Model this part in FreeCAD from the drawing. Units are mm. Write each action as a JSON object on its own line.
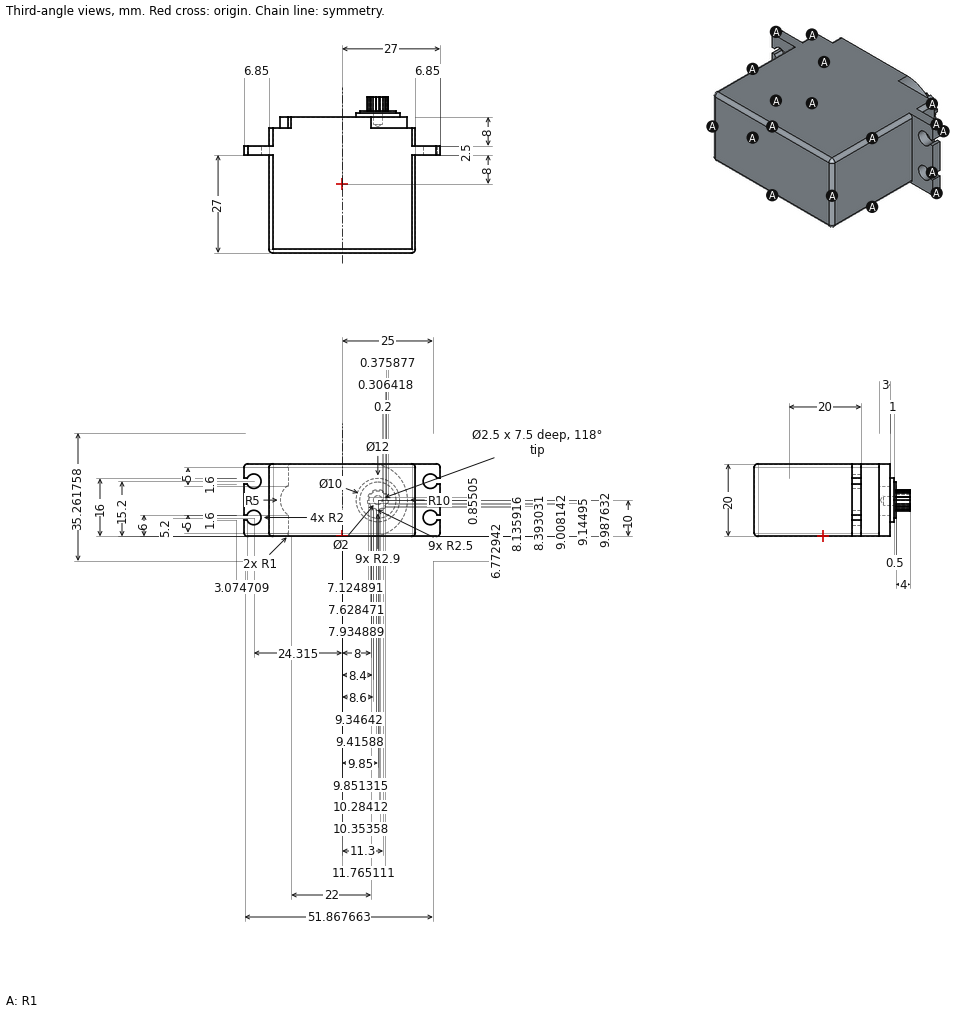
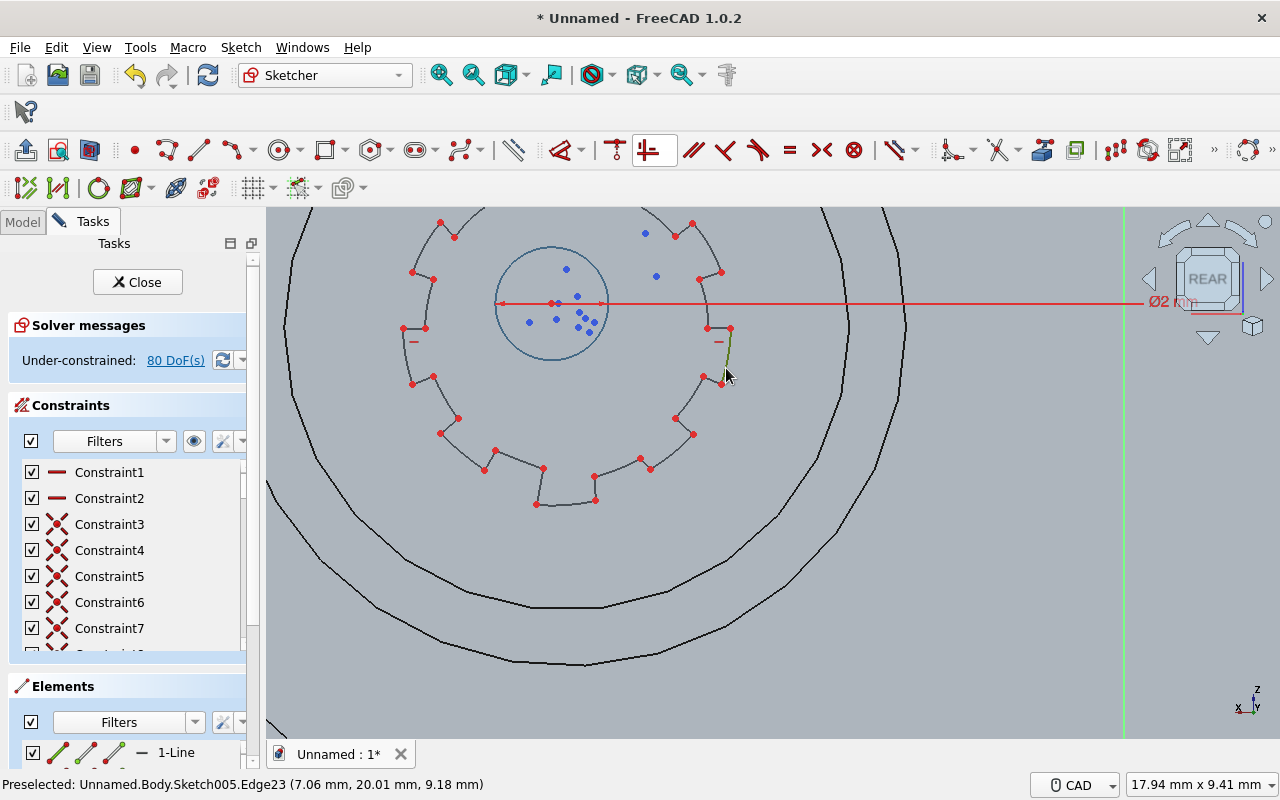
{"action": "left_click", "coordinate": [616, 150]}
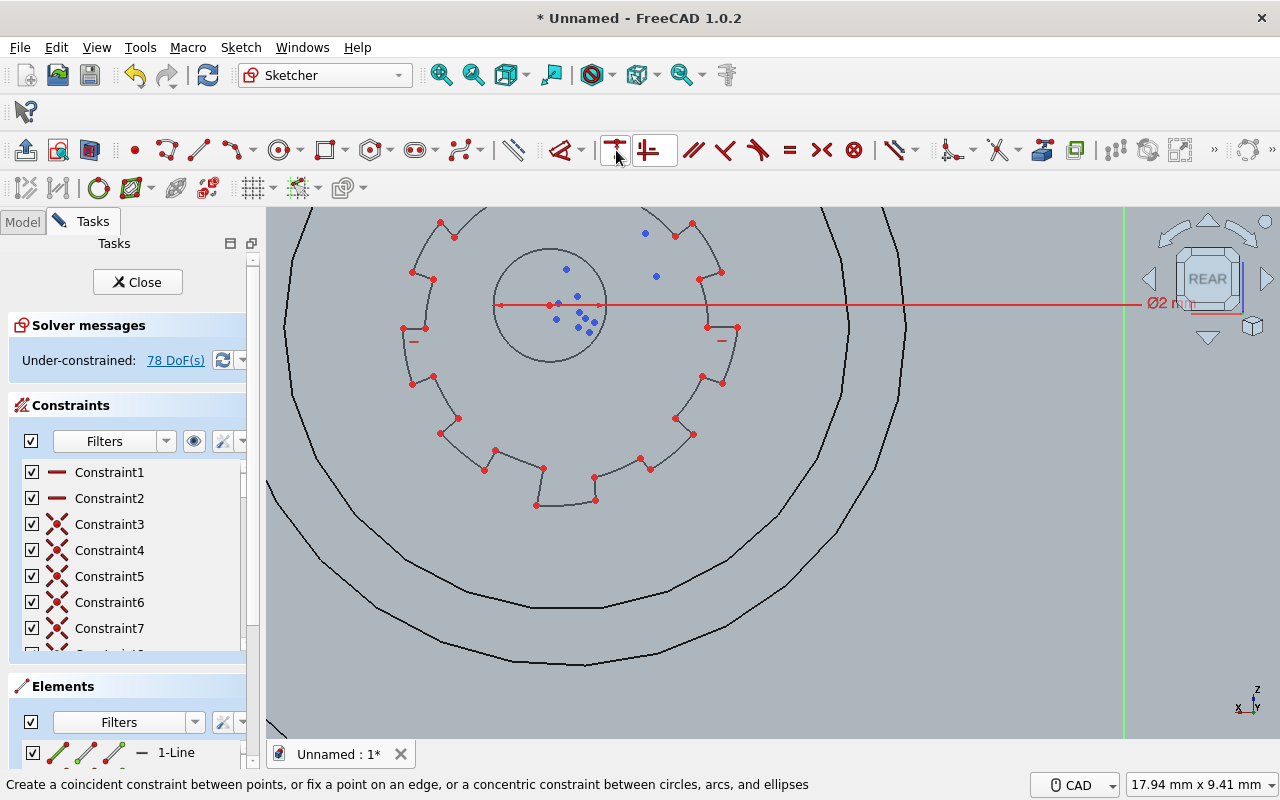
{"action": "left_click", "coordinate": [590, 265]}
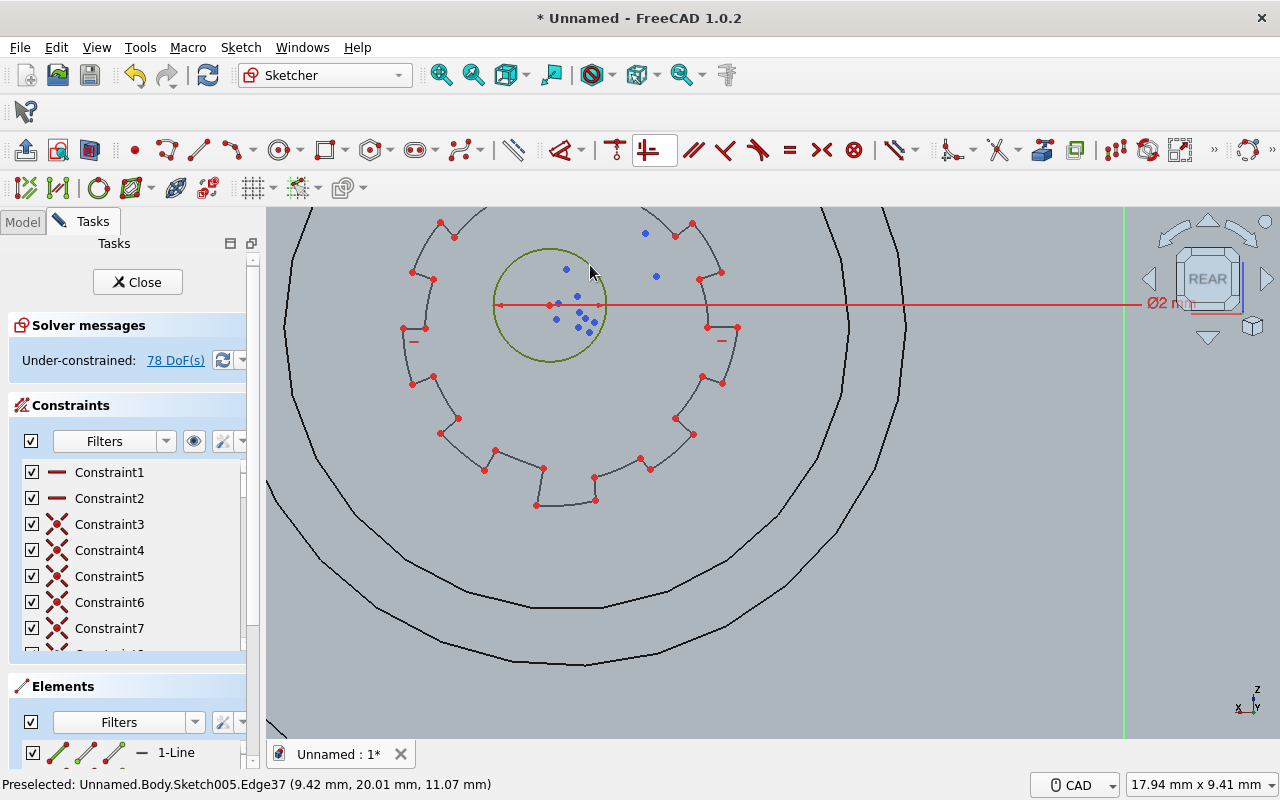
{"action": "left_click", "coordinate": [707, 313]}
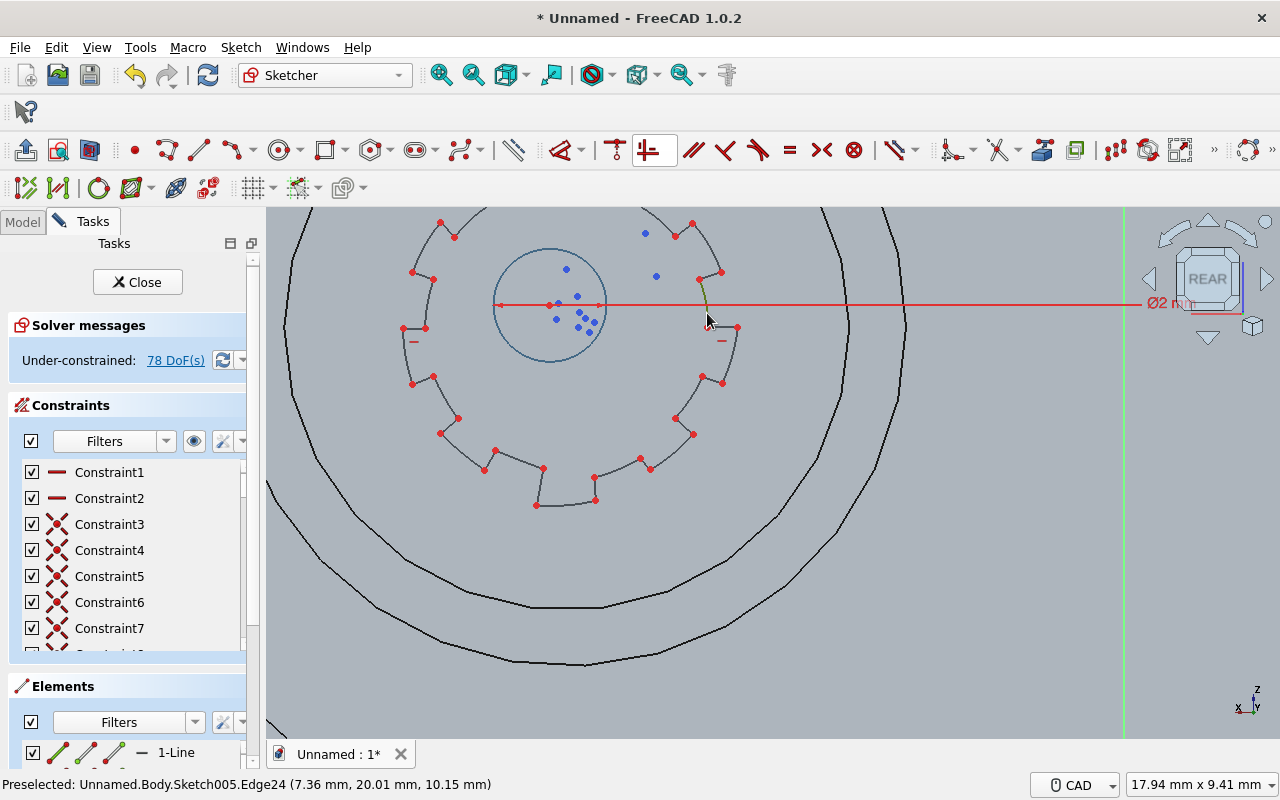
{"action": "left_click", "coordinate": [616, 150]}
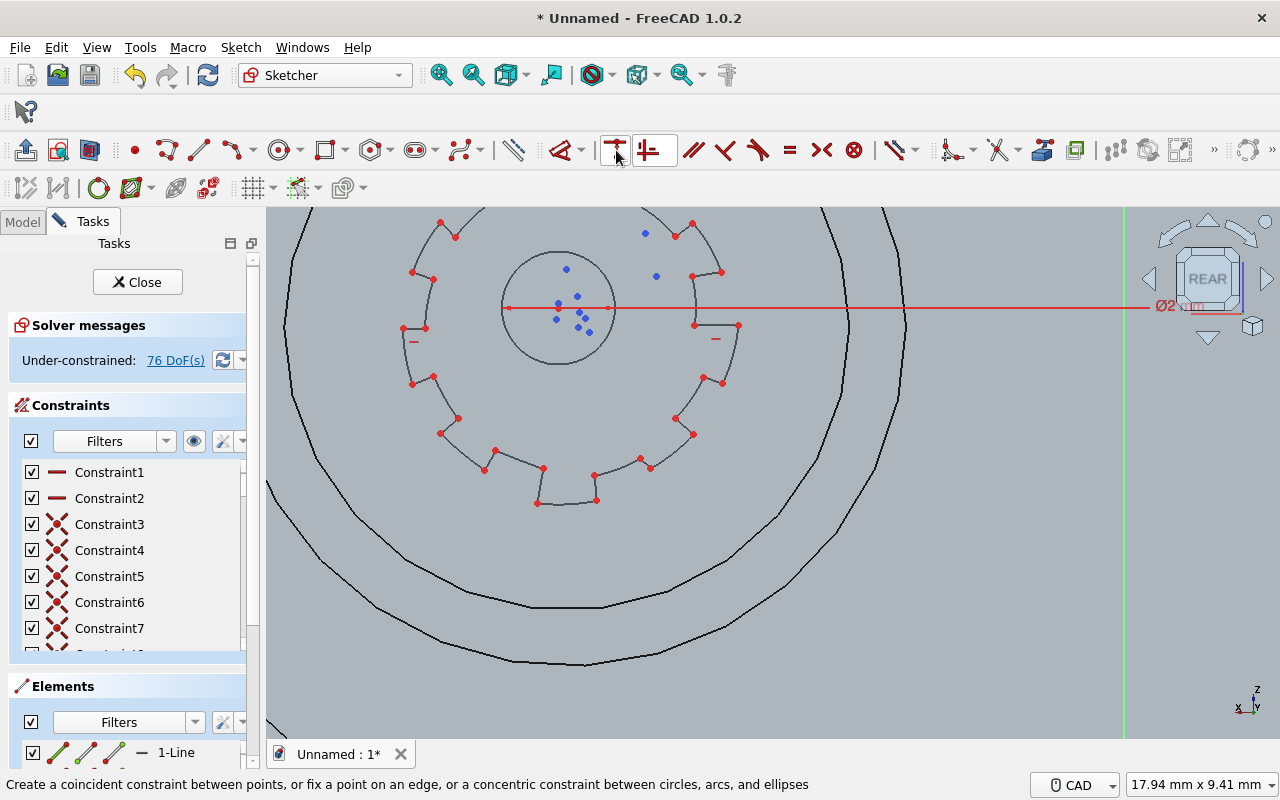
{"action": "left_click", "coordinate": [598, 268]}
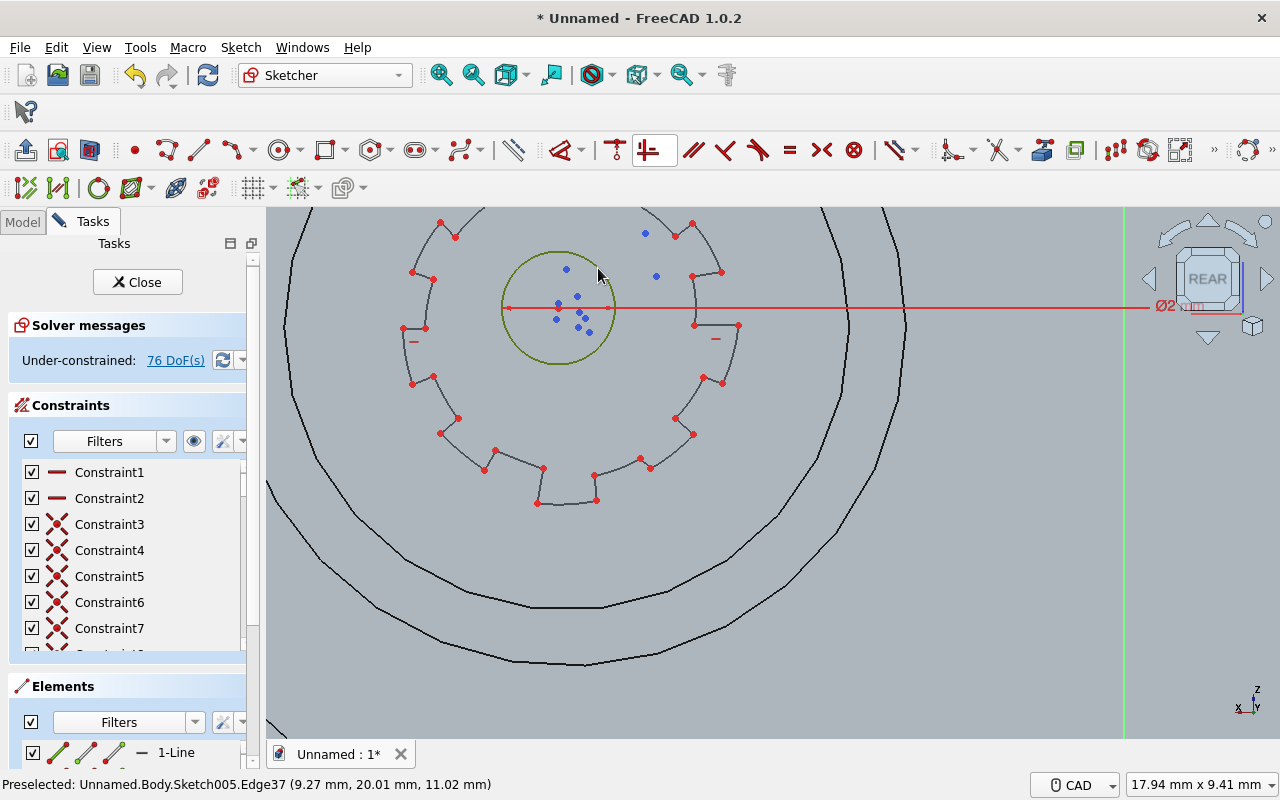
{"action": "left_click", "coordinate": [715, 256]}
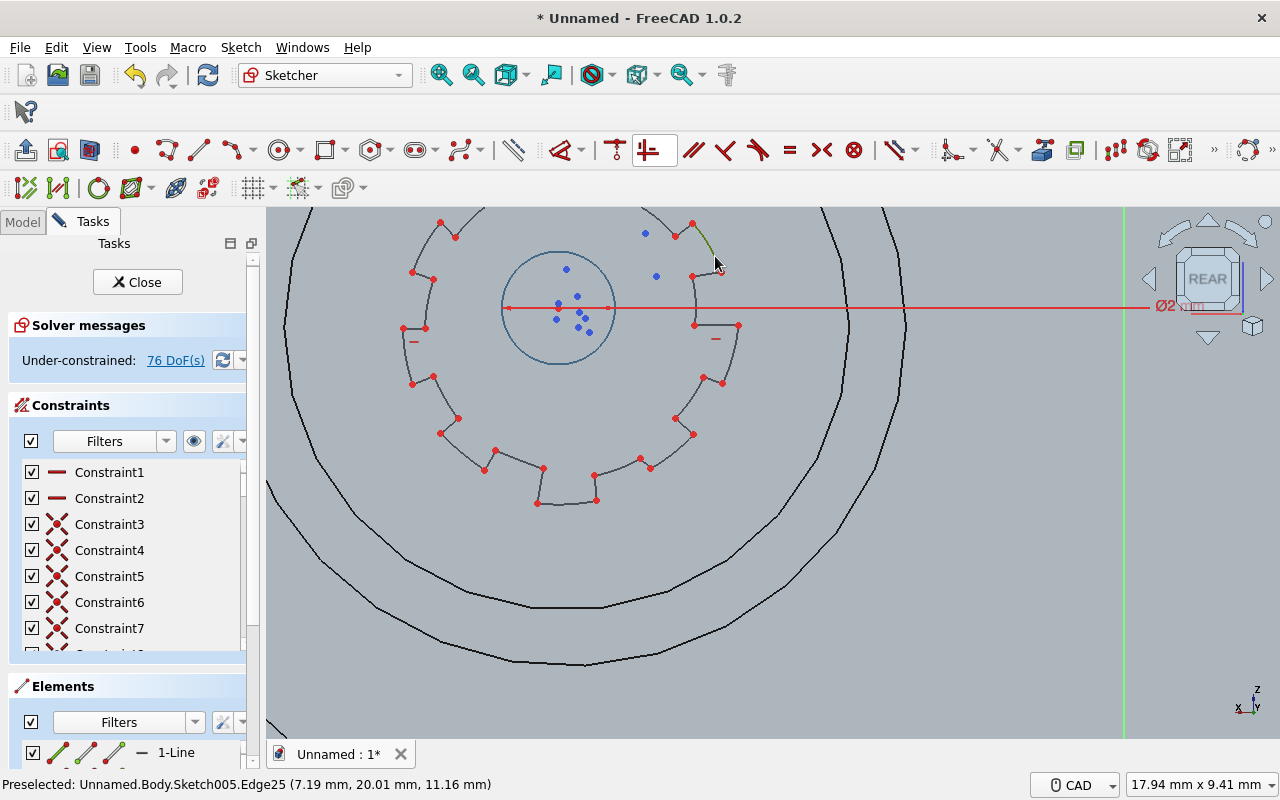
{"action": "left_click", "coordinate": [616, 150]}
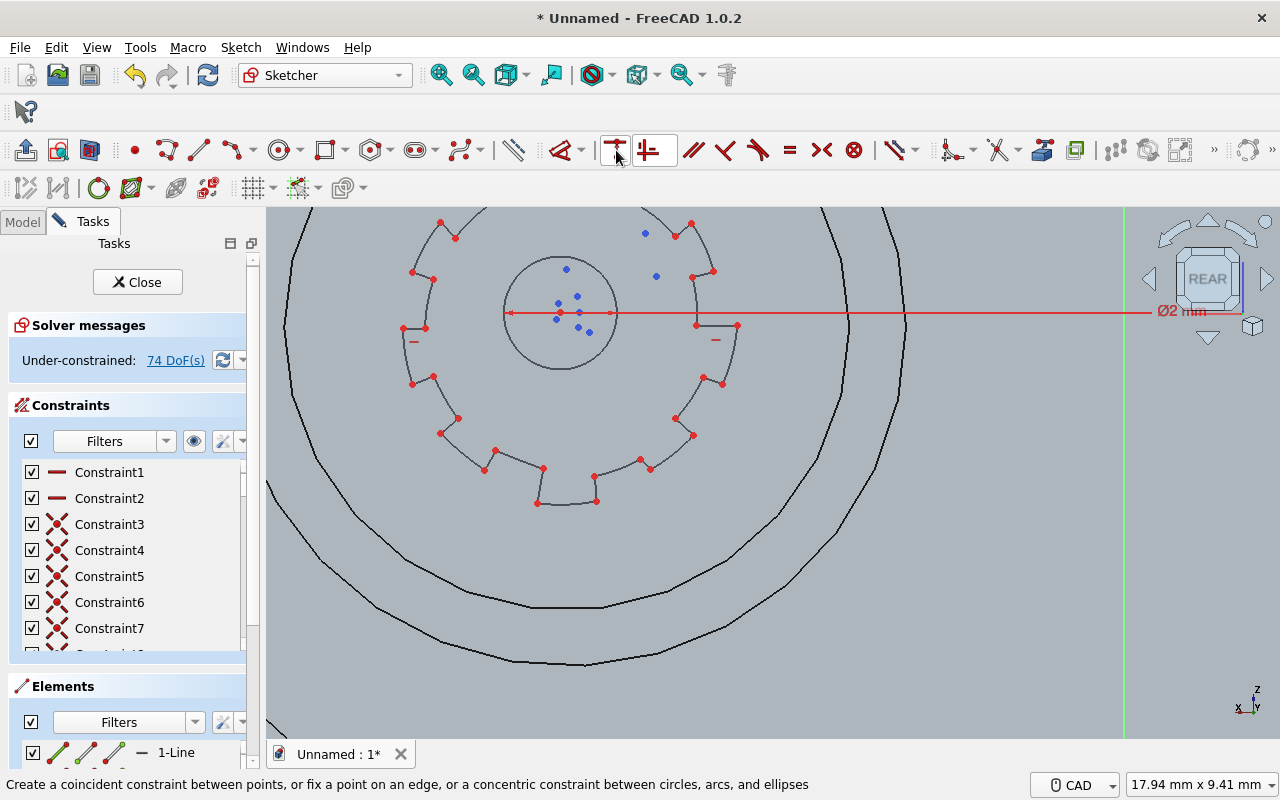
{"action": "left_click", "coordinate": [600, 273]}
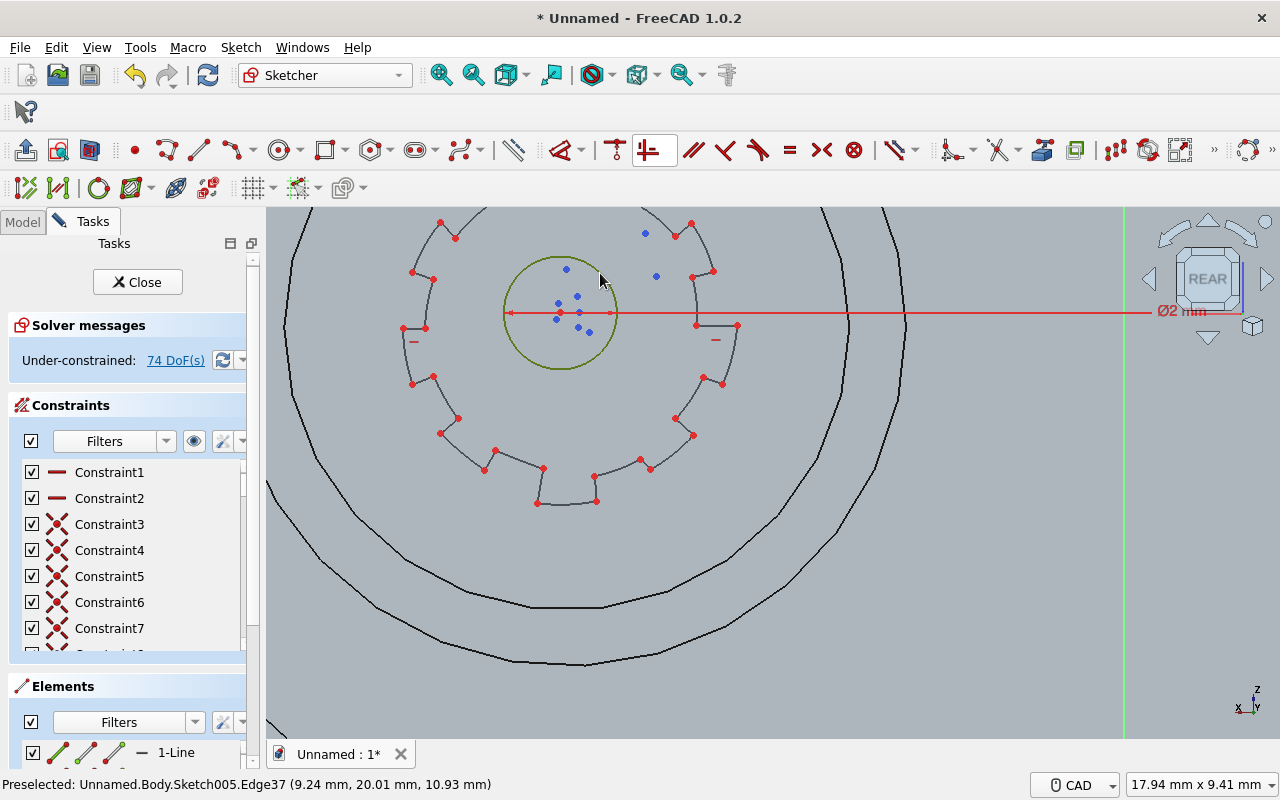
{"action": "scroll", "coordinate": [657, 427], "scroll_direction": "down", "scroll_amount": 4}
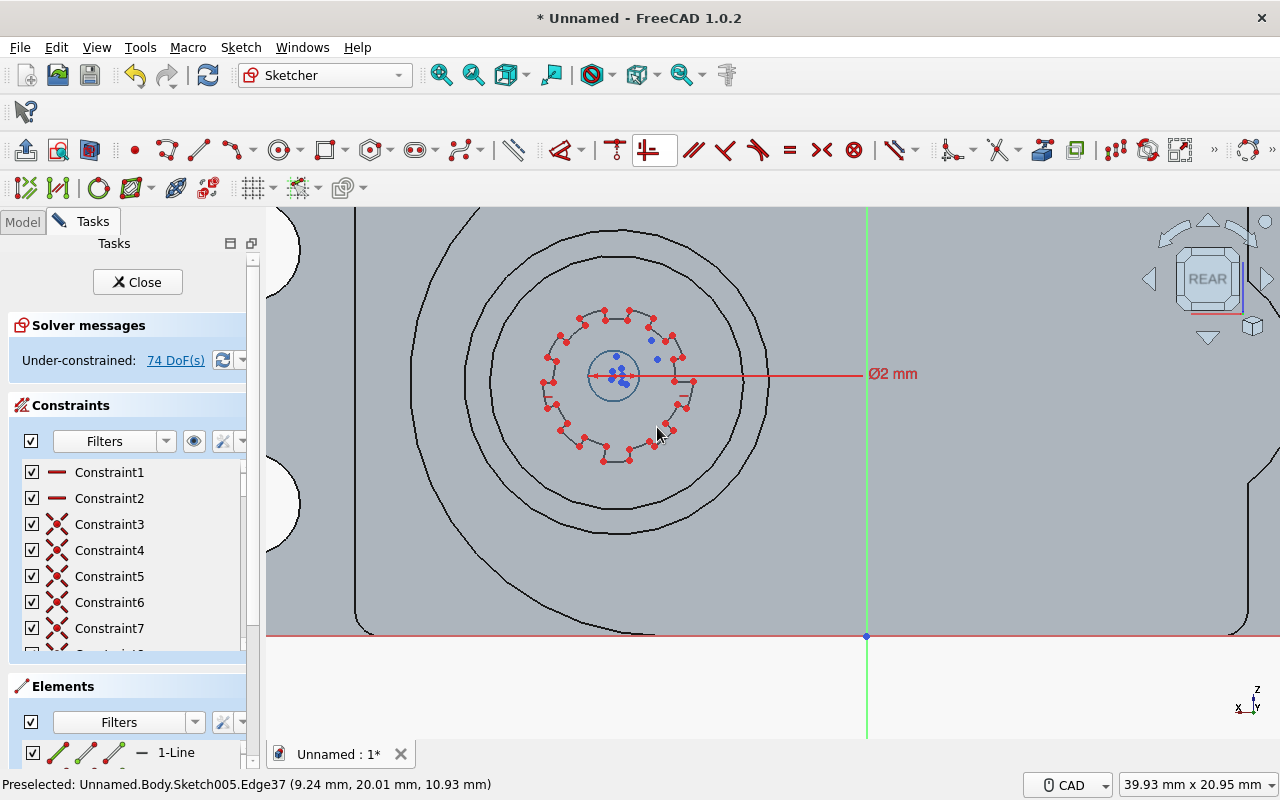
{"action": "scroll", "coordinate": [661, 337], "scroll_direction": "up", "scroll_amount": 4}